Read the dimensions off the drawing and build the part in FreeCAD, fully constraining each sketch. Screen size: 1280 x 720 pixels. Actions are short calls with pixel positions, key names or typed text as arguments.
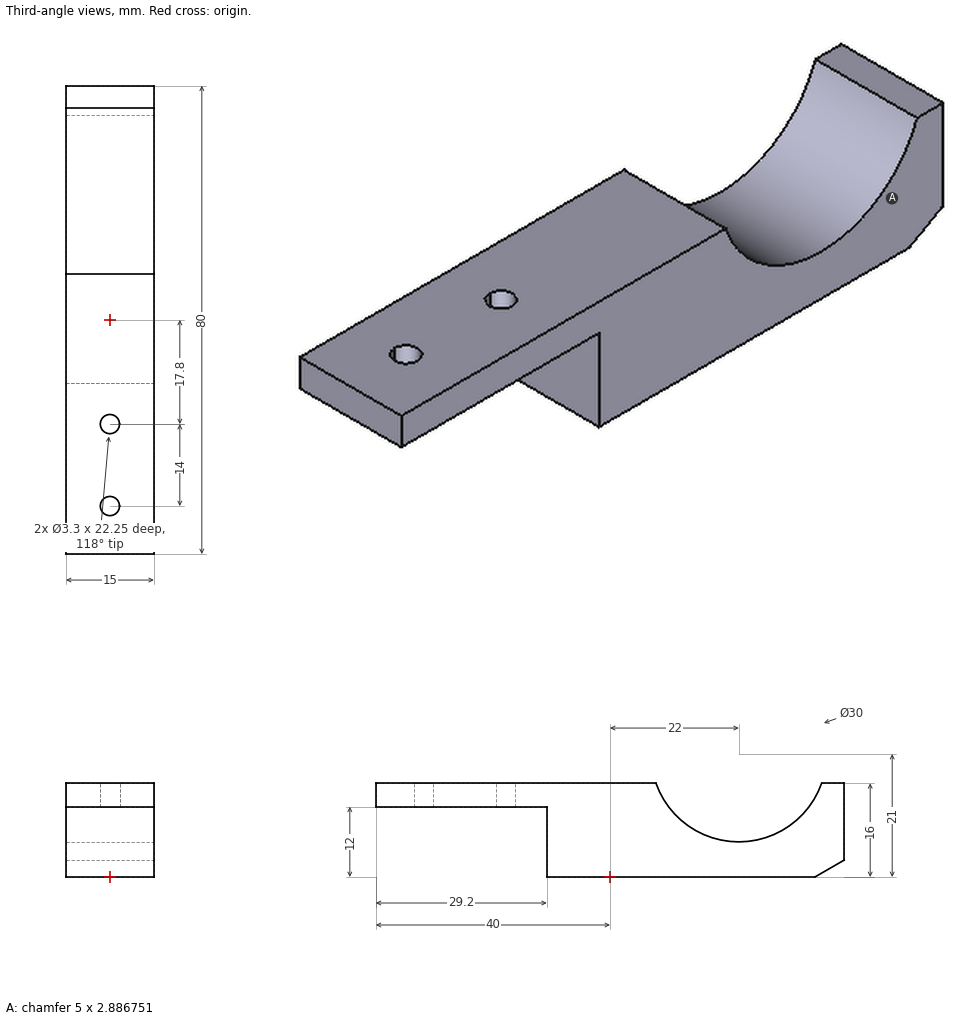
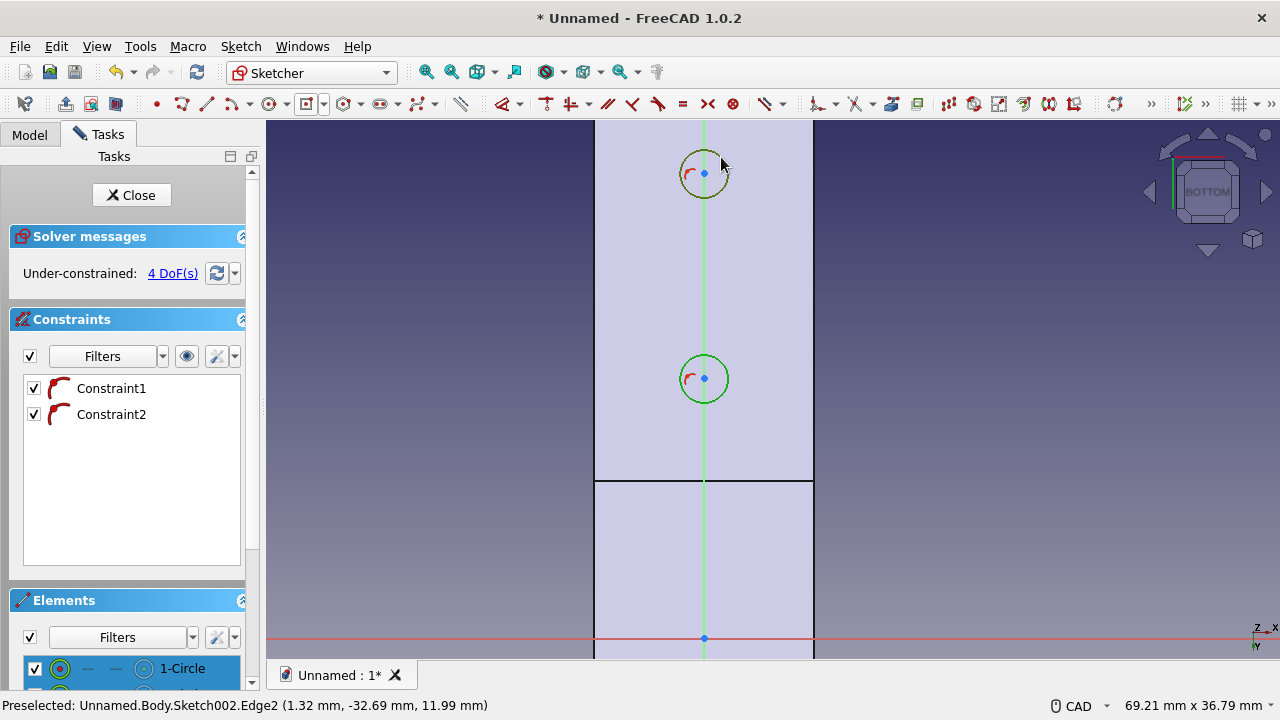
click(683, 104)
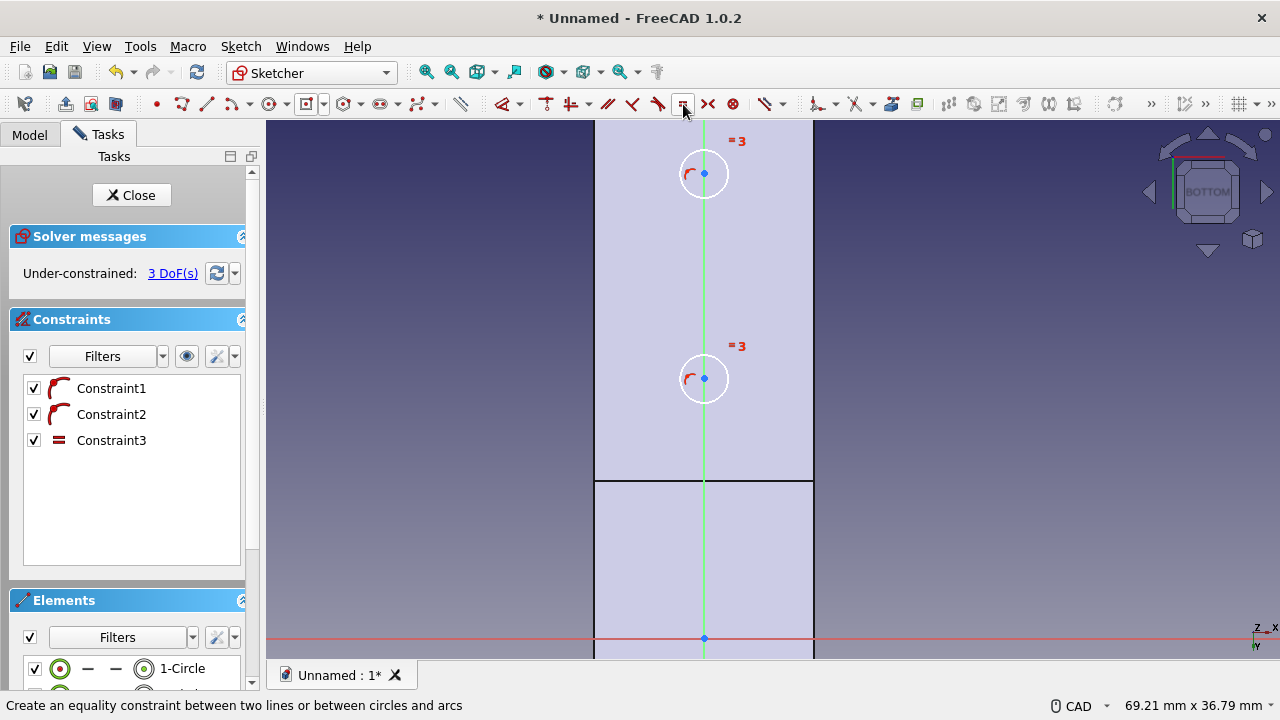
click(502, 104)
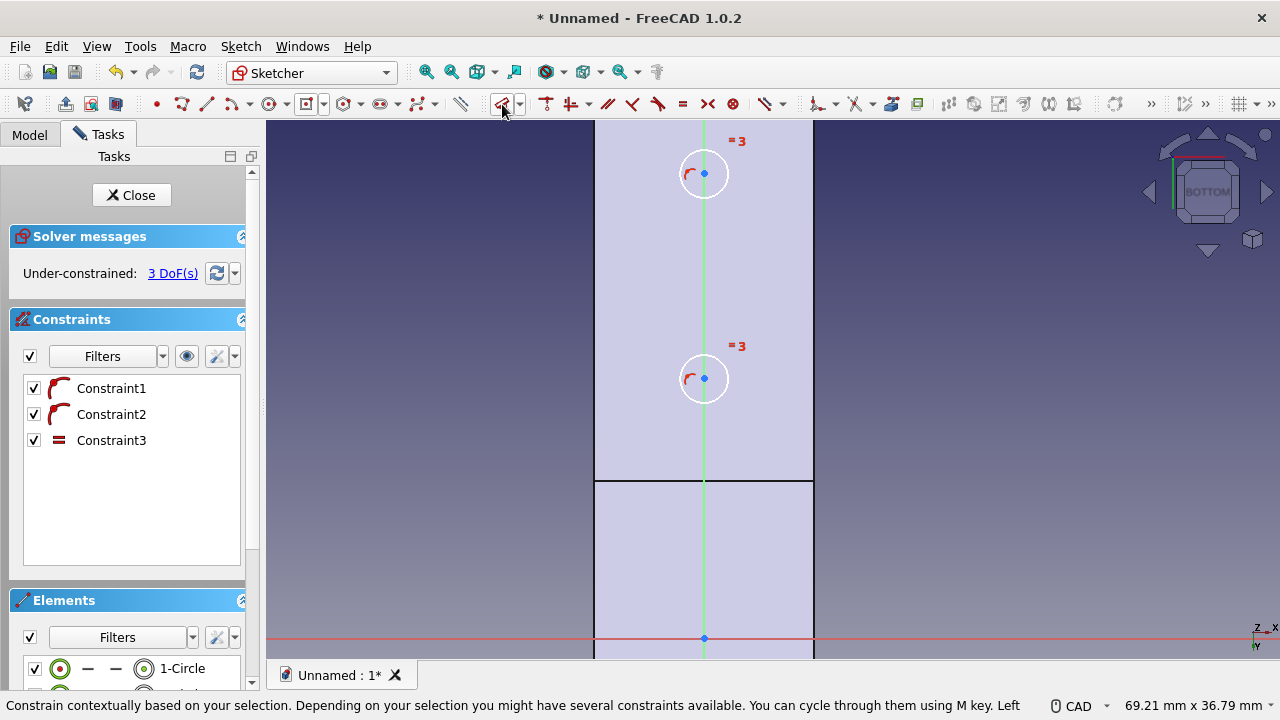
click(721, 362)
click(743, 339)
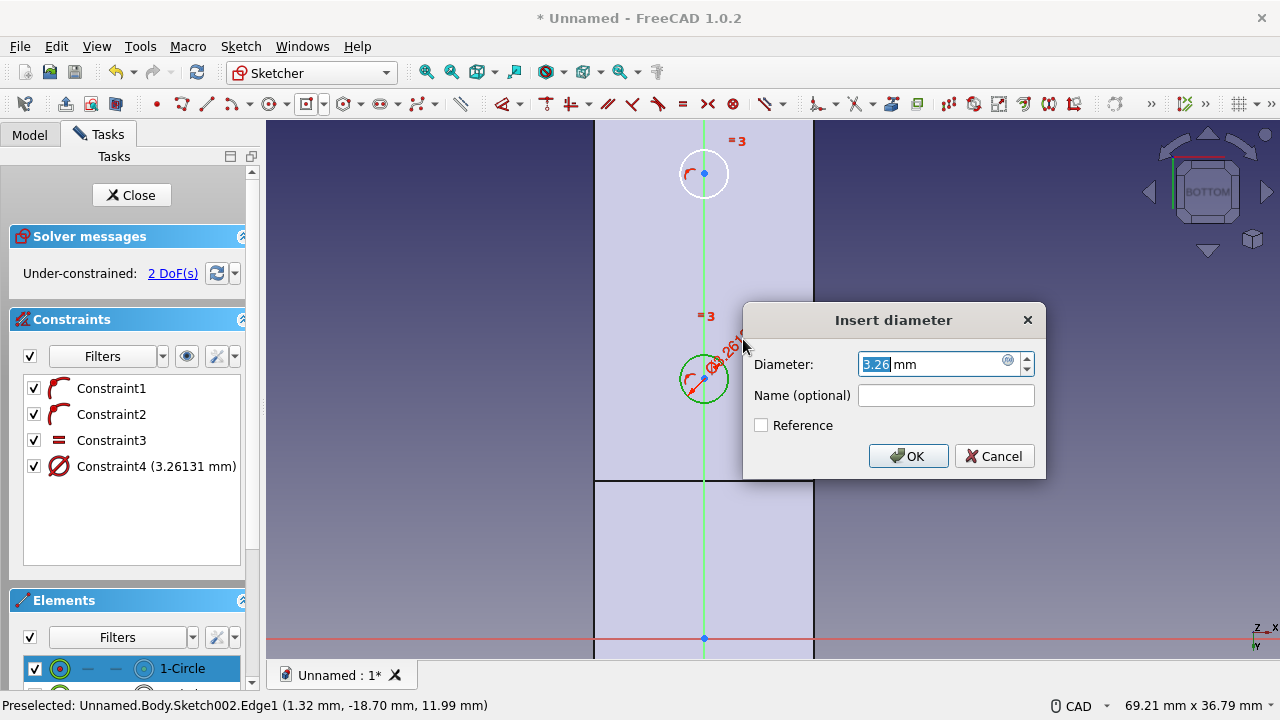
text(3.3)
key(Return)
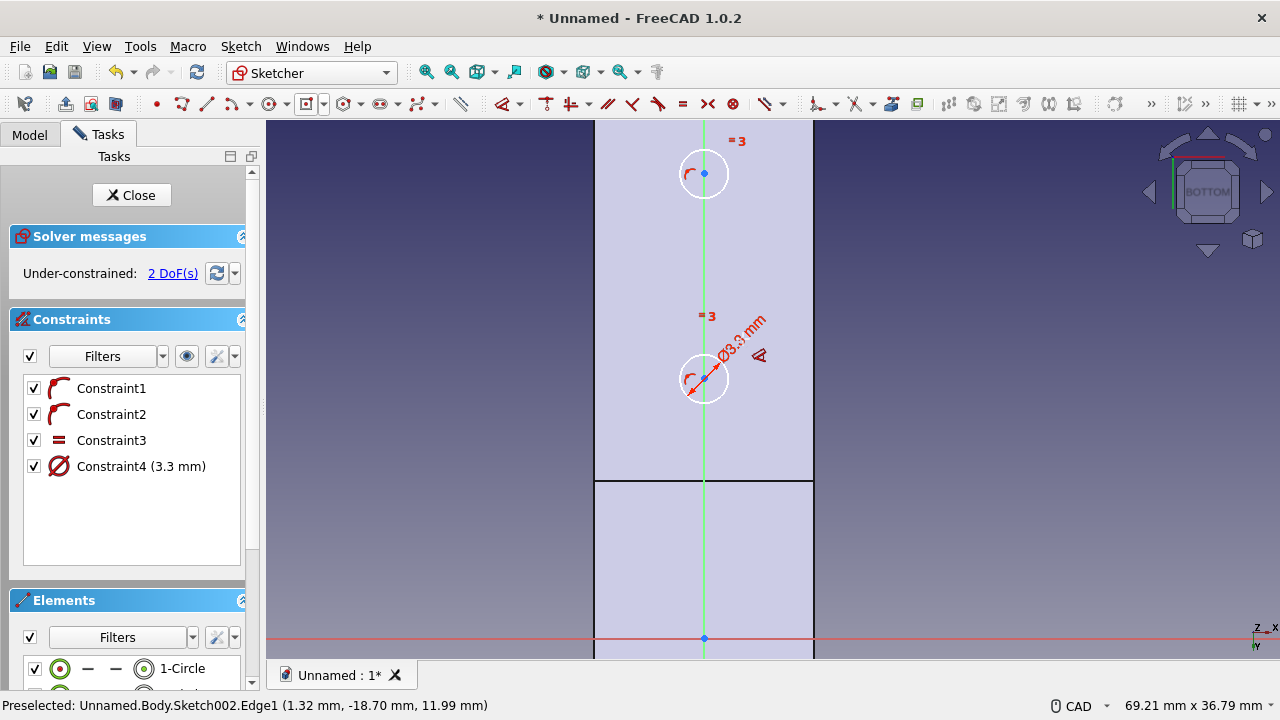
click(704, 379)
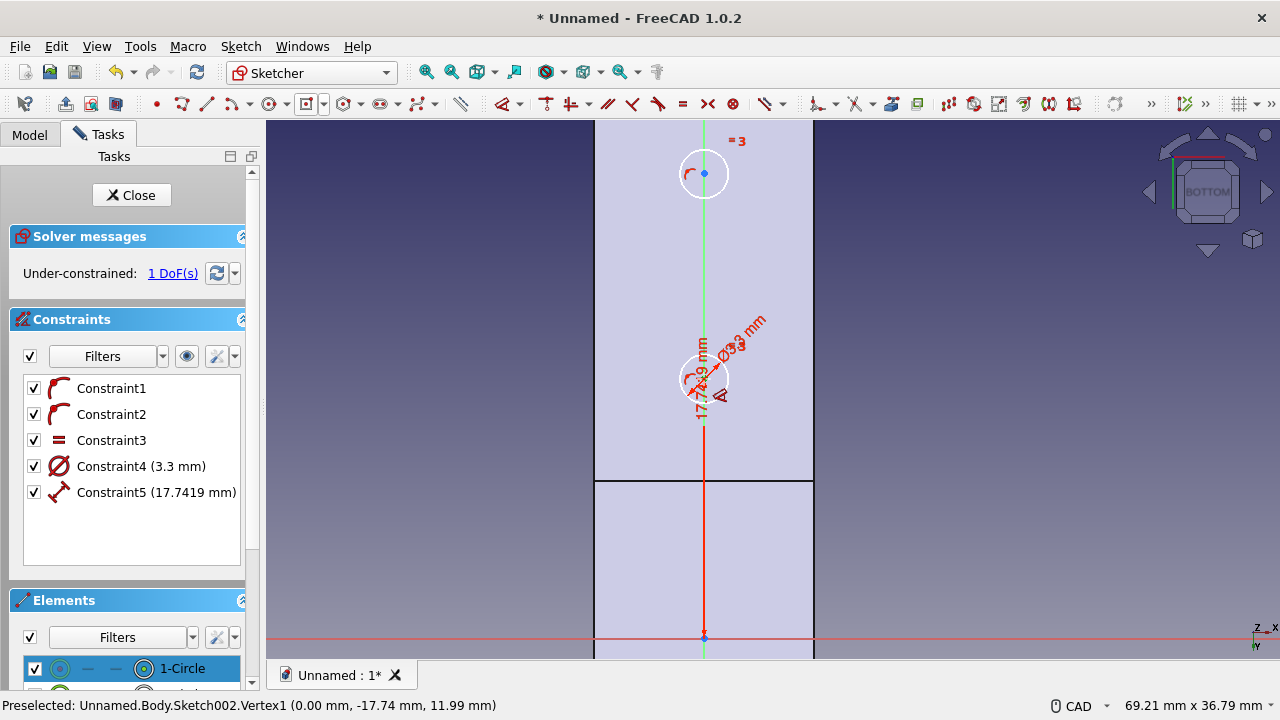
click(704, 174)
click(738, 276)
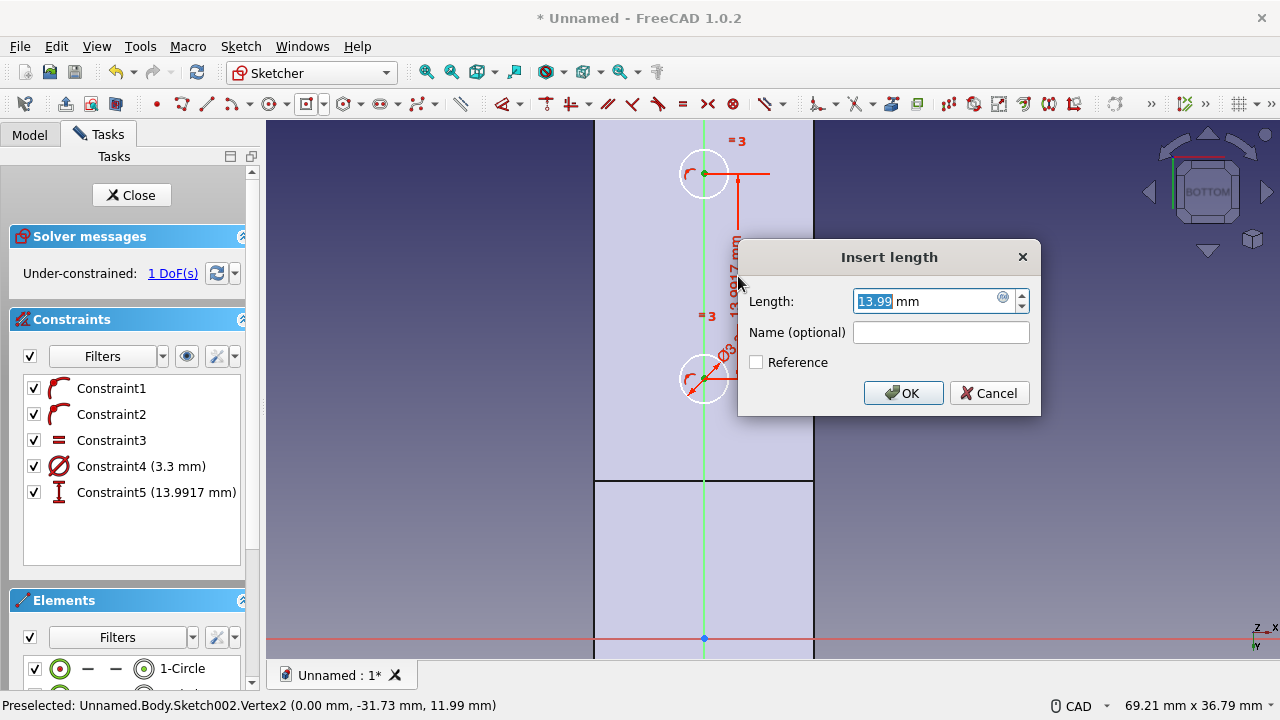
text(14)
key(Return)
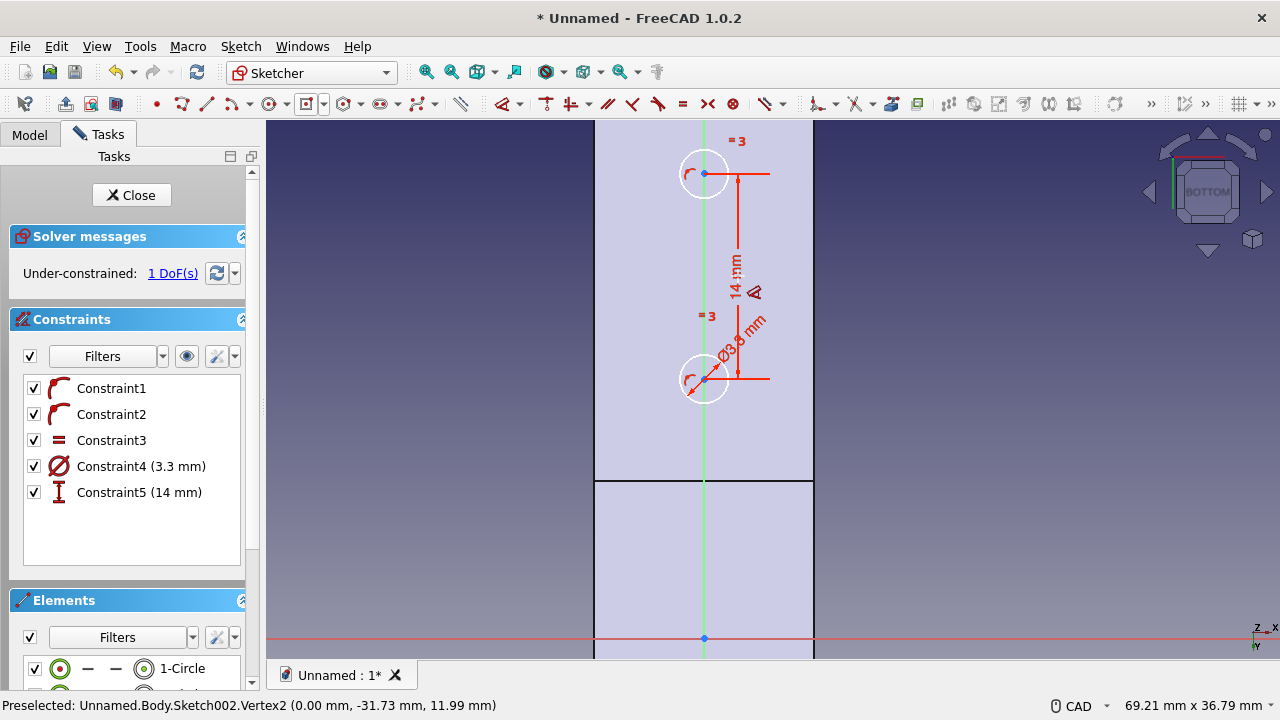
click(704, 379)
click(738, 505)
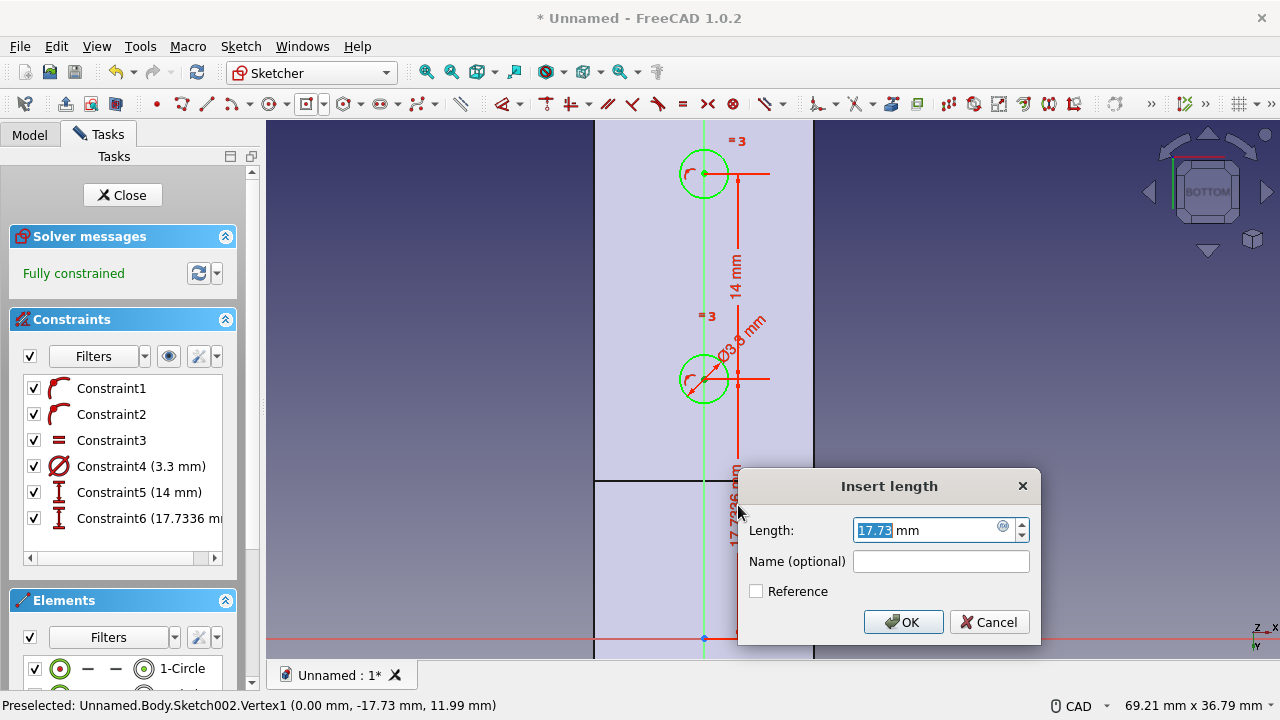
text(17.8)
key(Return)
key(Escape)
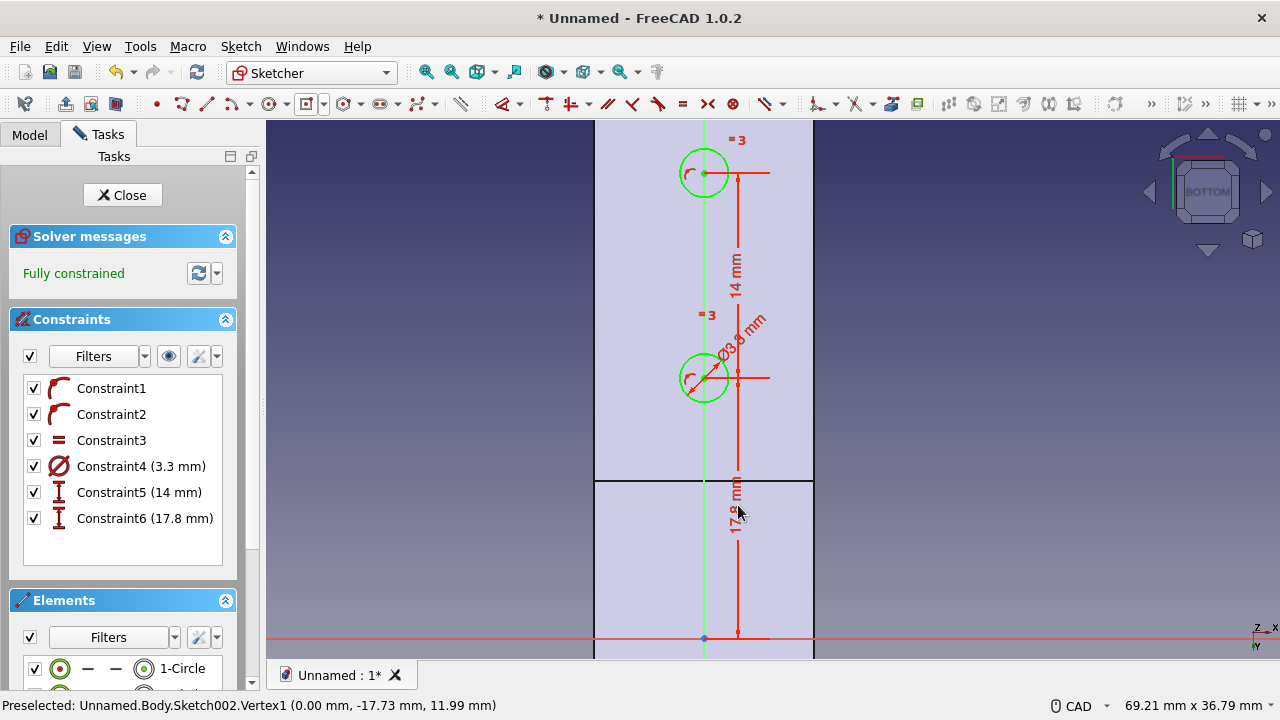
click(123, 195)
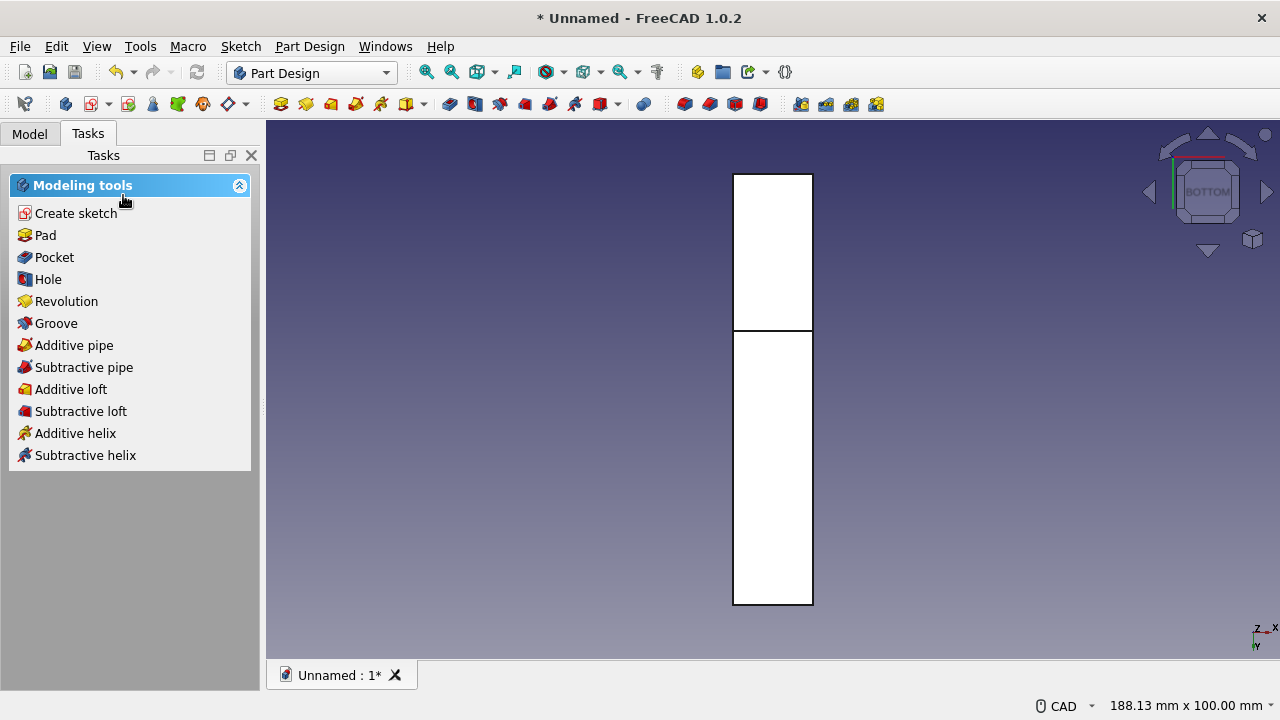
click(475, 104)